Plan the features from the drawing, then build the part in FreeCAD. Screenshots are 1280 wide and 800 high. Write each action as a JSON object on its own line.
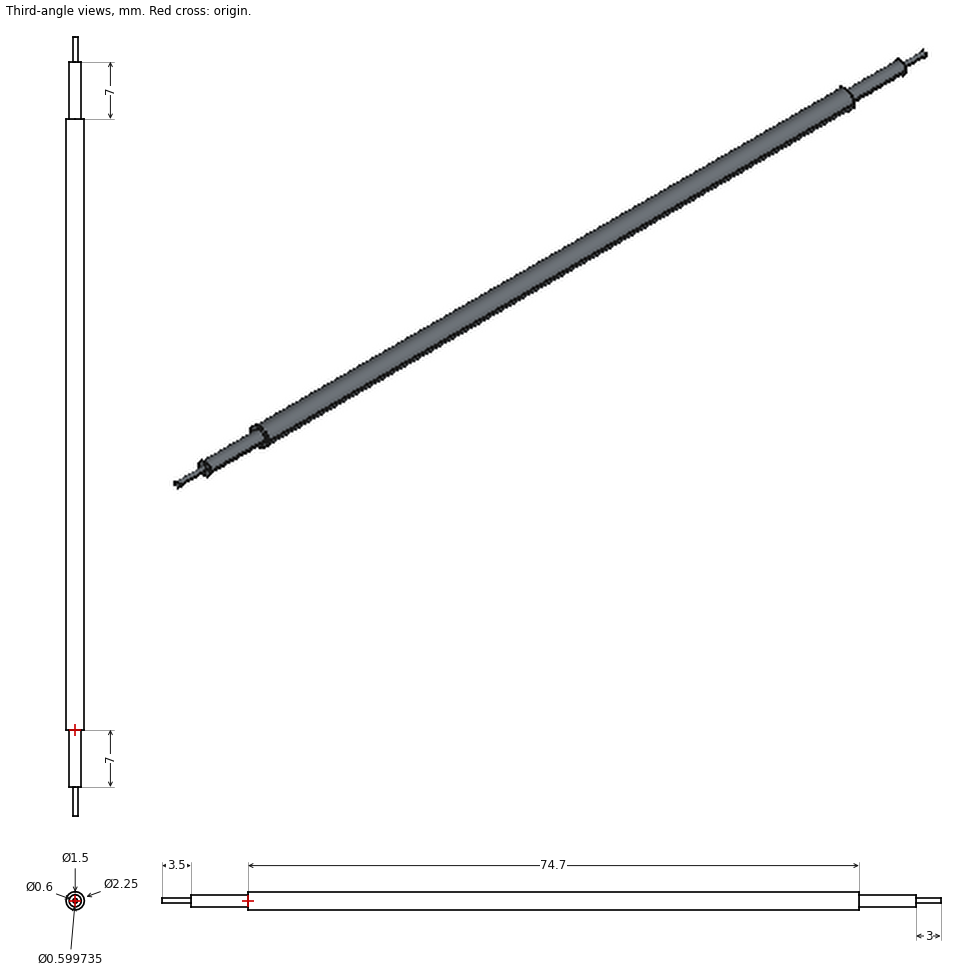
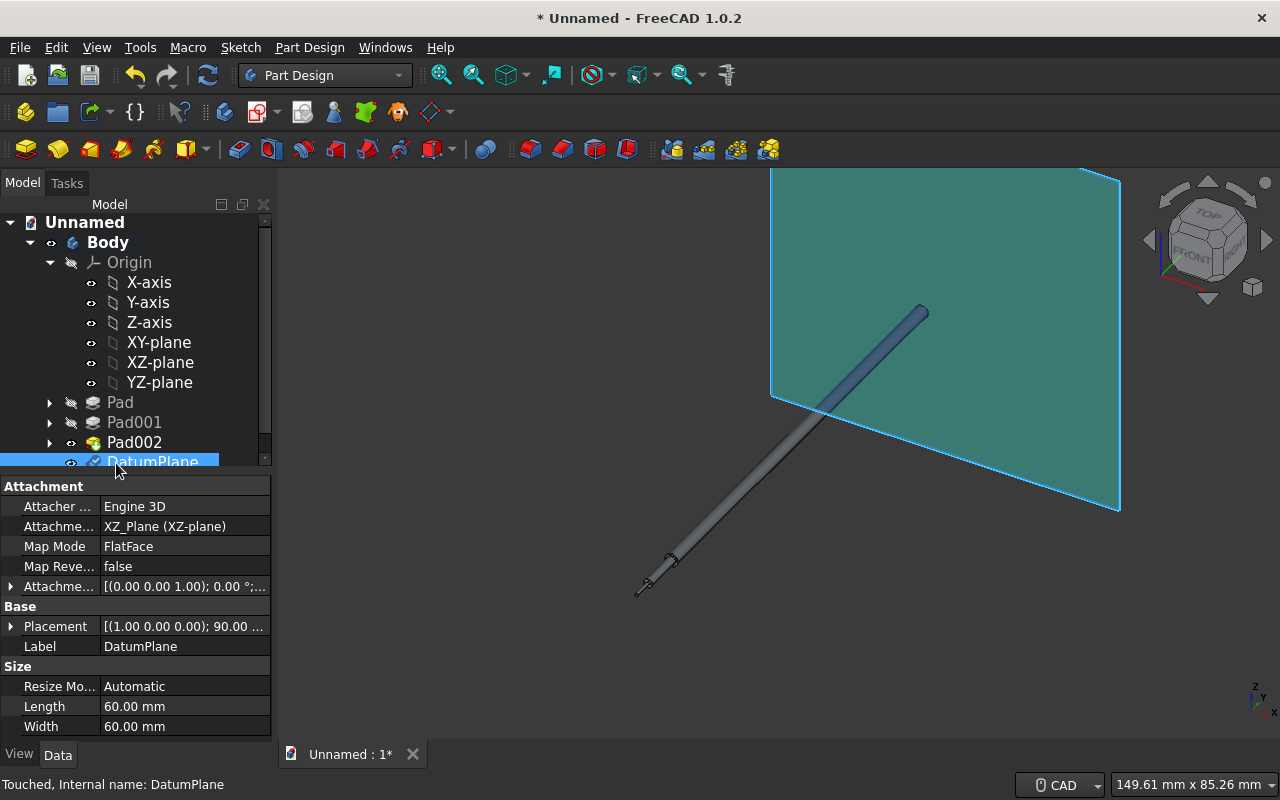
{"action": "left_click", "coordinate": [258, 112]}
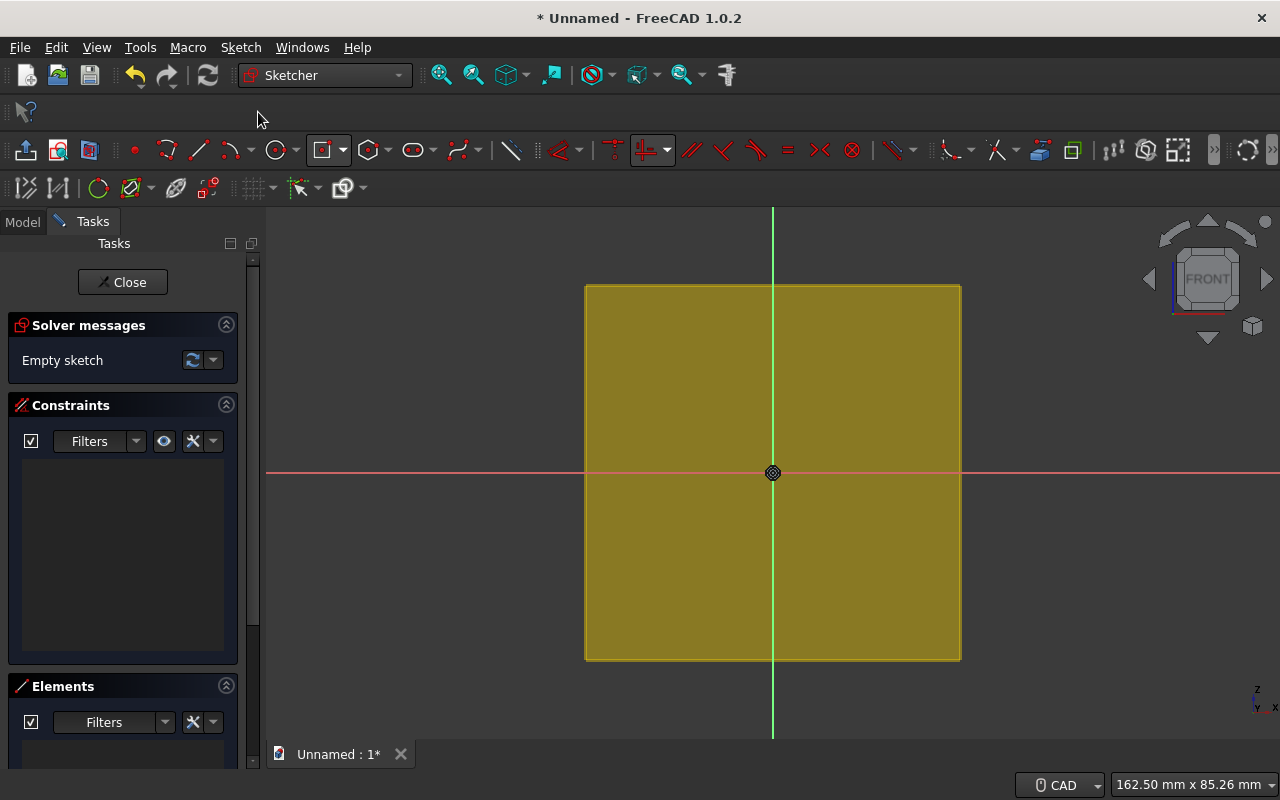
{"action": "left_click", "coordinate": [90, 150]}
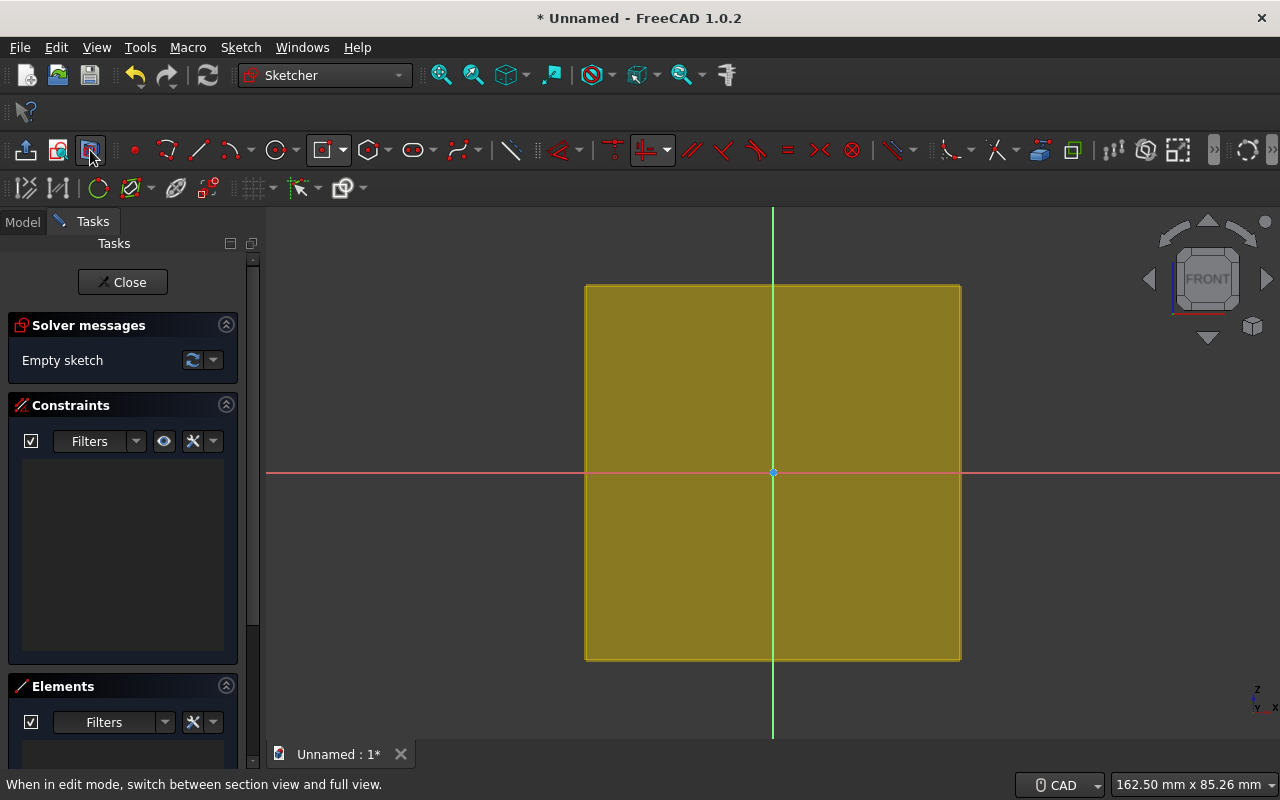
{"action": "scroll", "coordinate": [777, 473], "scroll_direction": "up", "scroll_amount": 15}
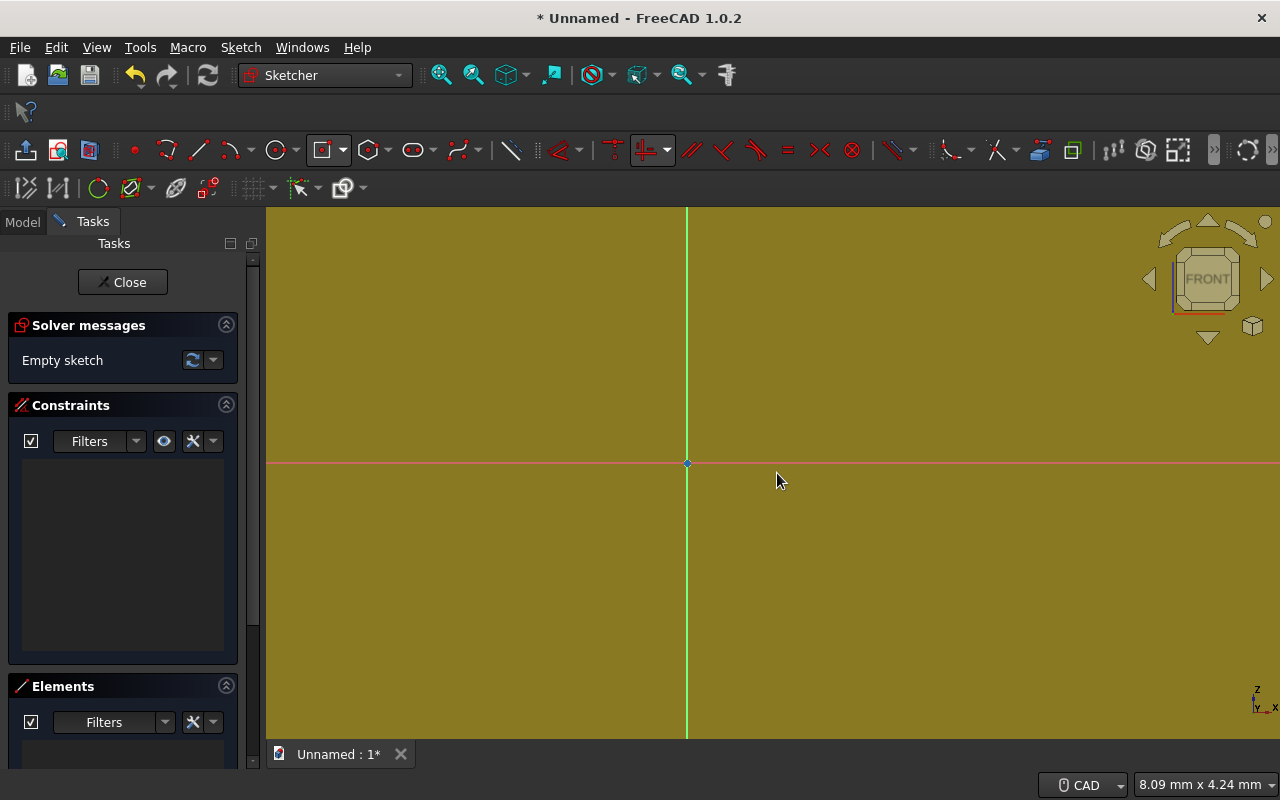
{"action": "scroll", "coordinate": [666, 452], "scroll_direction": "up", "scroll_amount": 3}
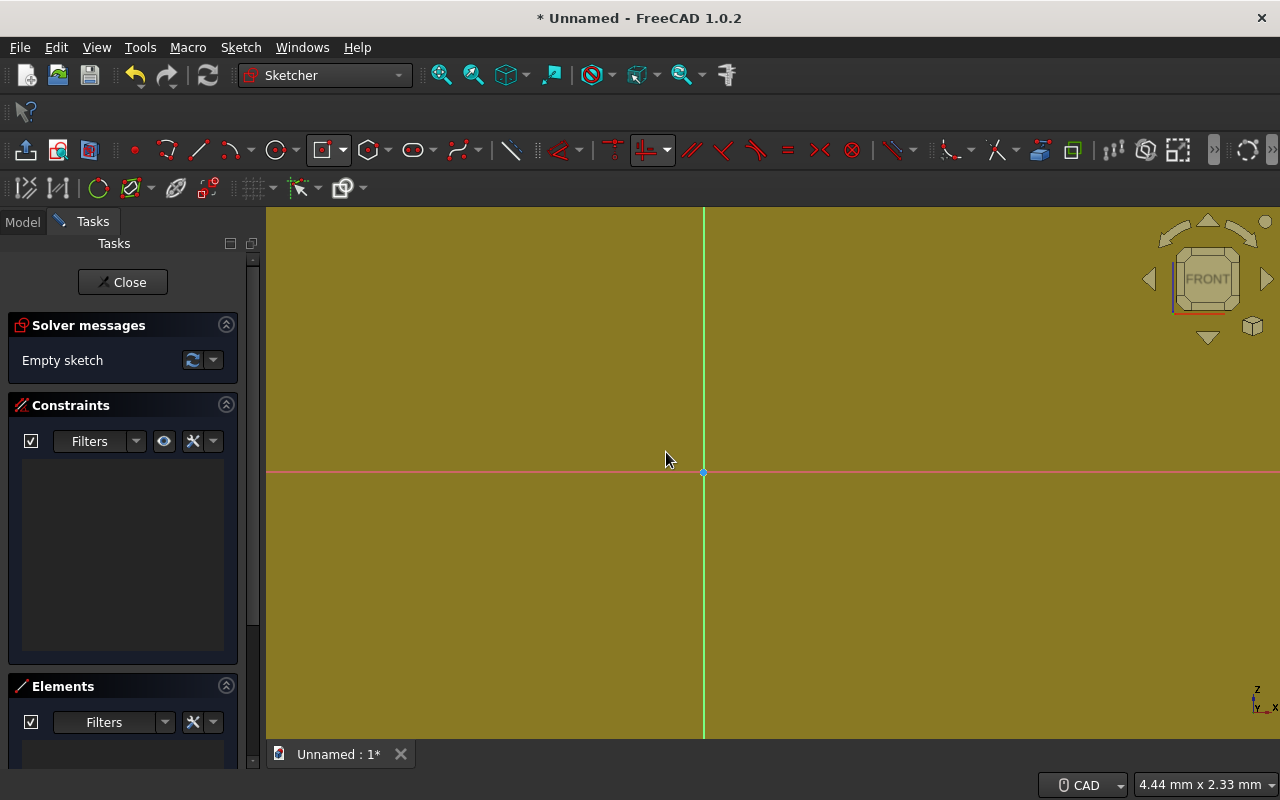
{"action": "left_click", "coordinate": [276, 150]}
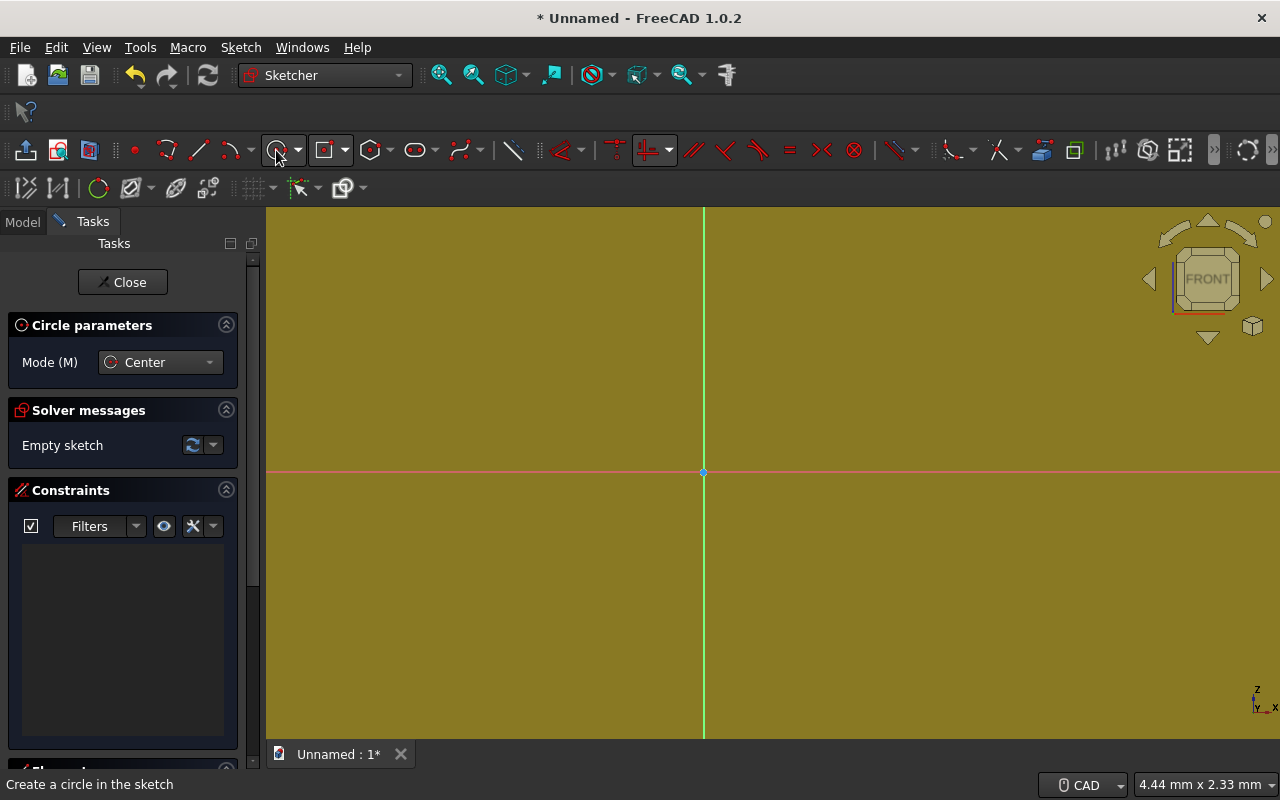
{"action": "left_click", "coordinate": [704, 472]}
{"action": "mouse_move", "coordinate": [825, 351]}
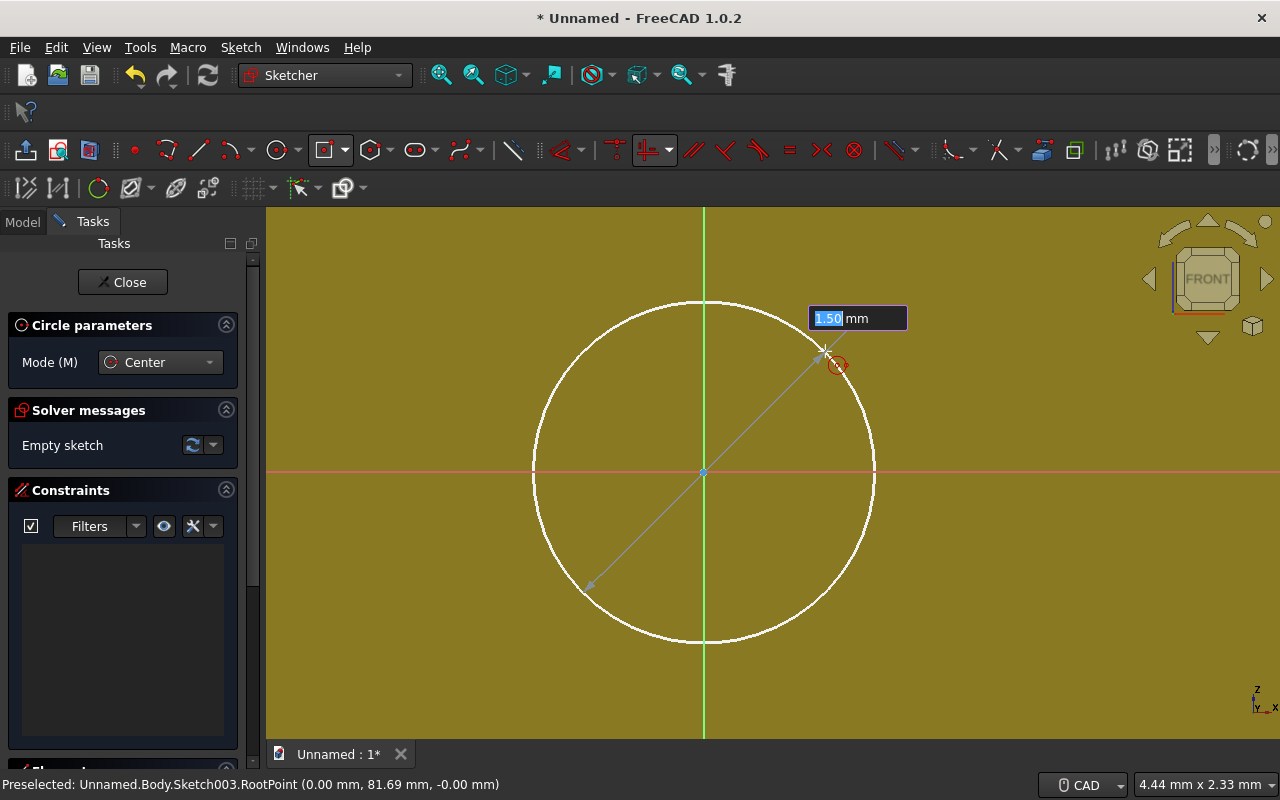
{"action": "type", "text": "1.5"}
{"action": "key", "text": "Return"}
{"action": "key", "text": "Escape"}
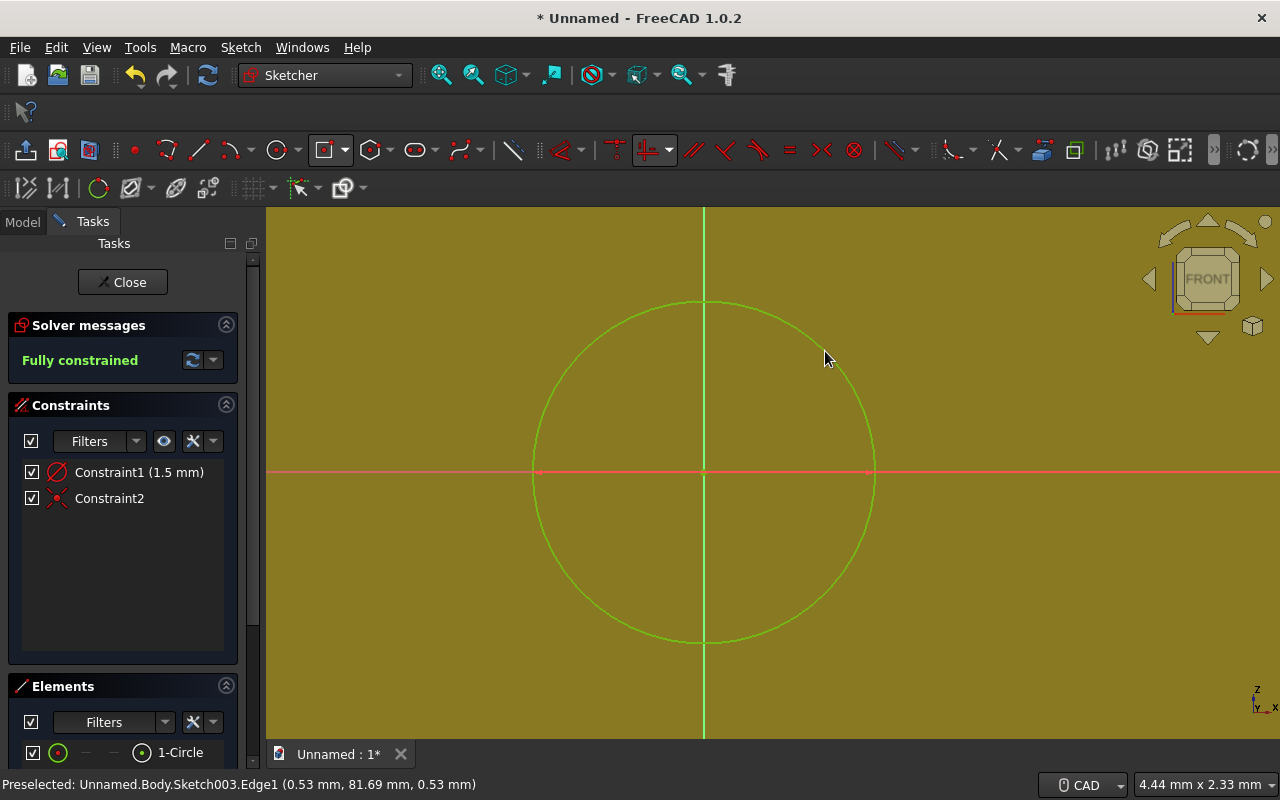
{"action": "left_click", "coordinate": [123, 282]}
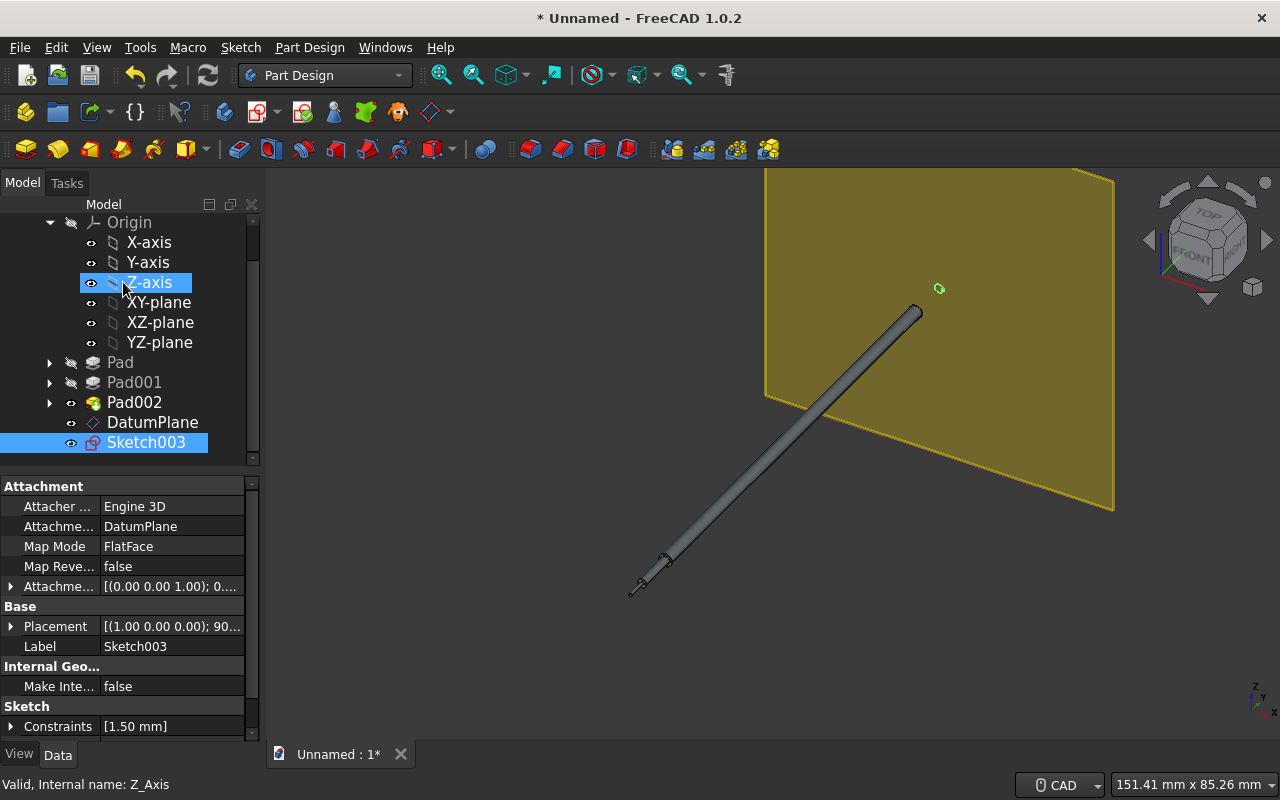
{"action": "left_click", "coordinate": [26, 150]}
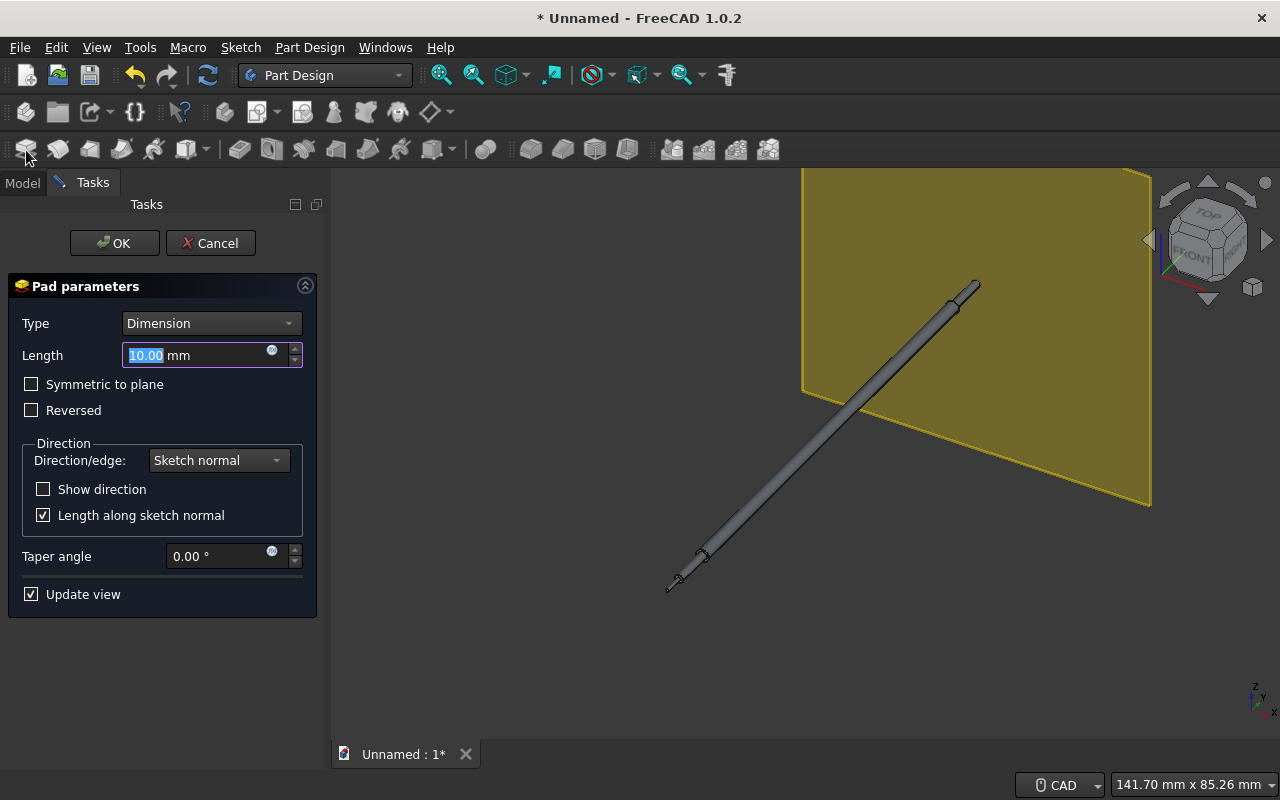
{"action": "type", "text": "7"}
{"action": "key", "text": "Tab"}